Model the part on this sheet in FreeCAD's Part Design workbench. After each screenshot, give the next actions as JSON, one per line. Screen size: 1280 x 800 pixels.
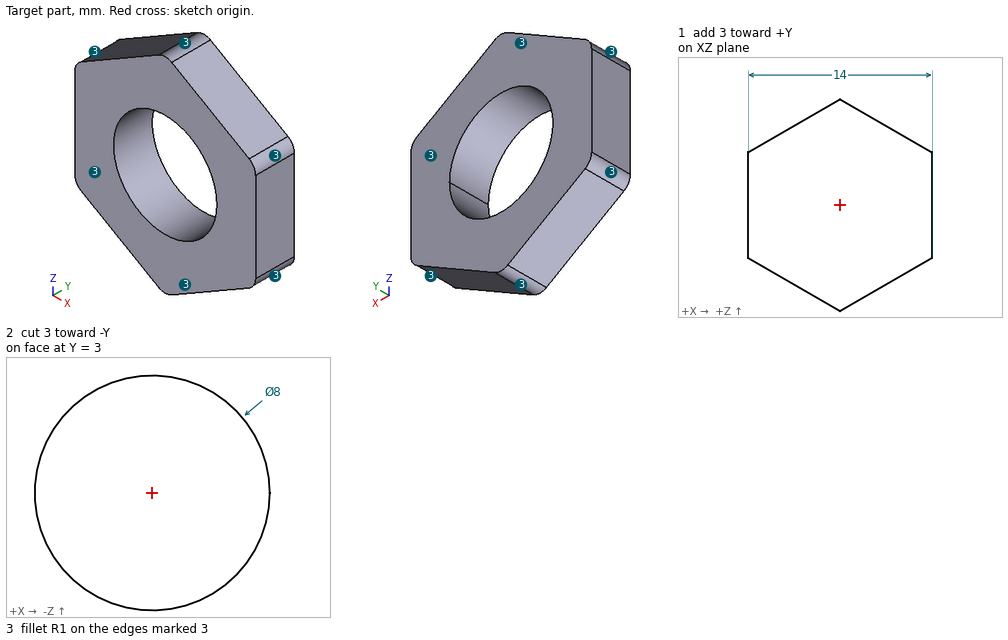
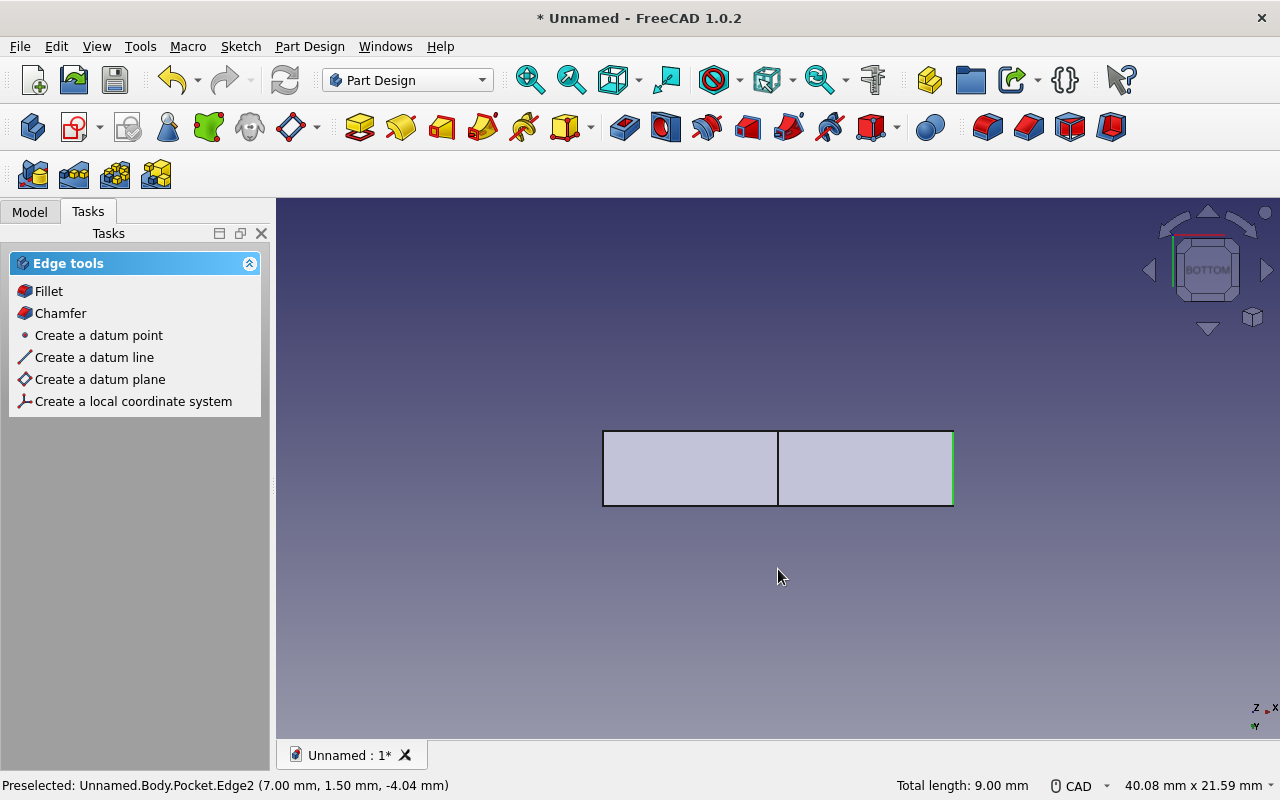
{"action": "key", "text": "v f"}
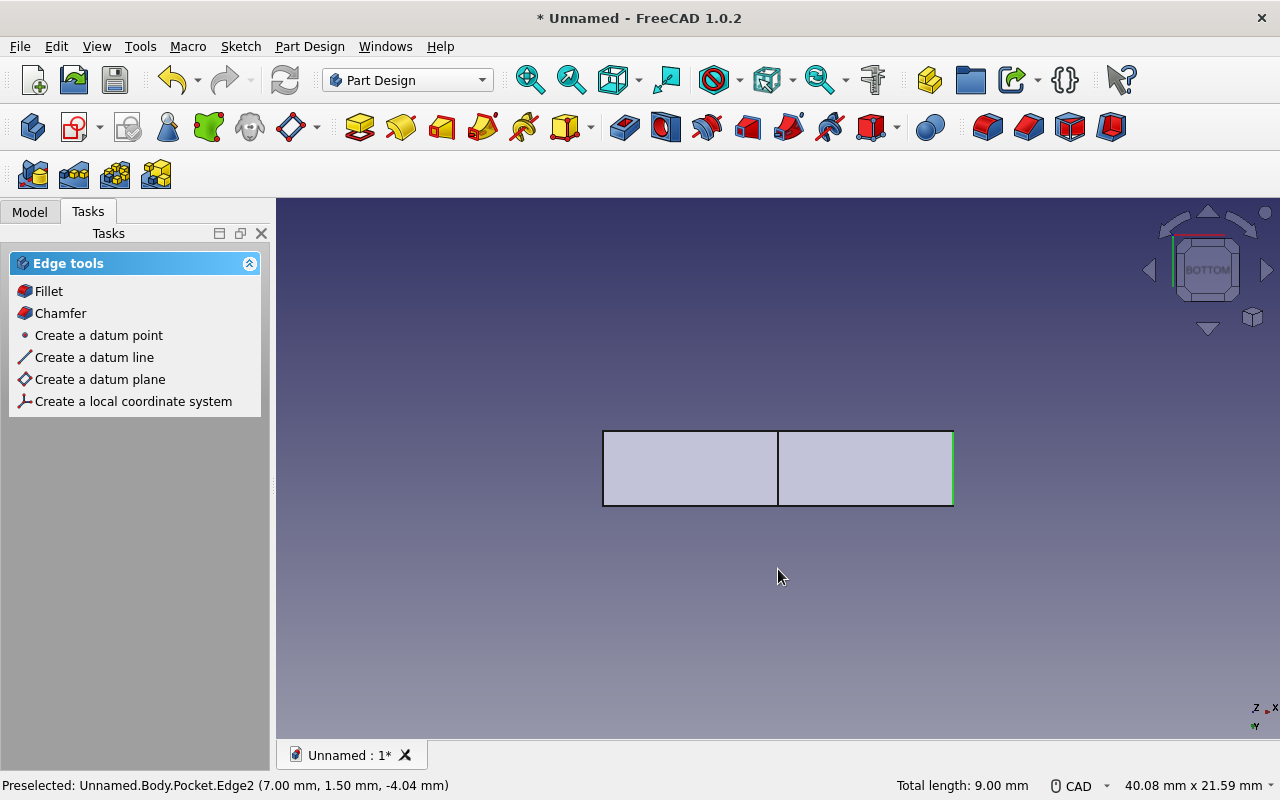
{"action": "left_click", "coordinate": [778, 467], "text": "ctrl"}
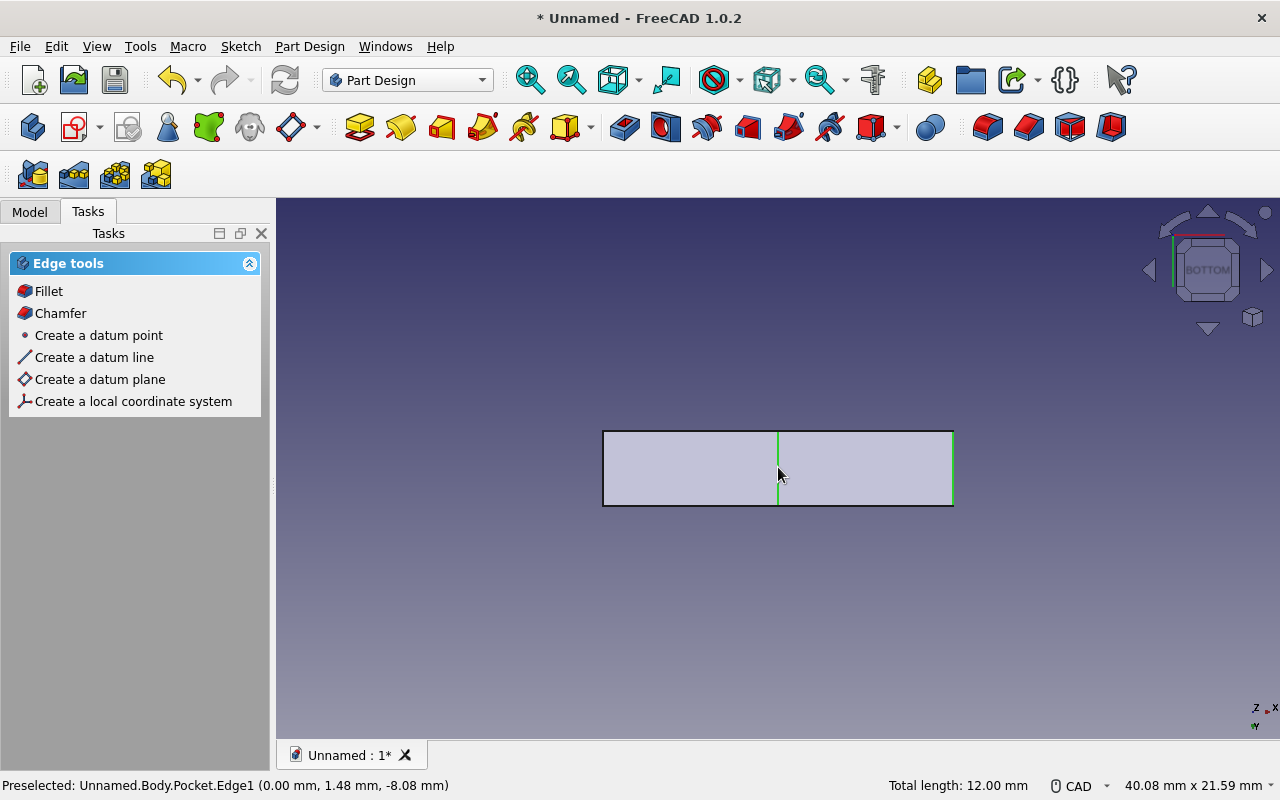
{"action": "key", "text": "4"}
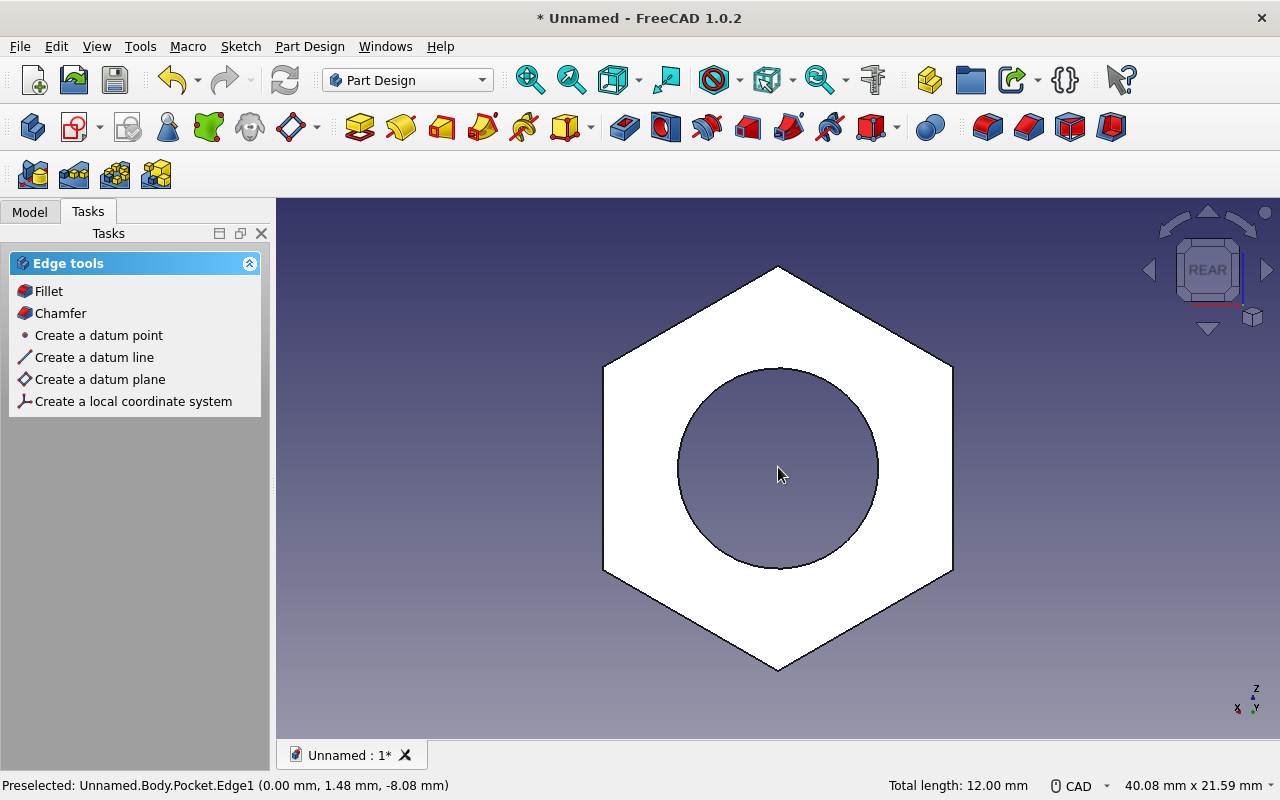
{"action": "key", "text": "6"}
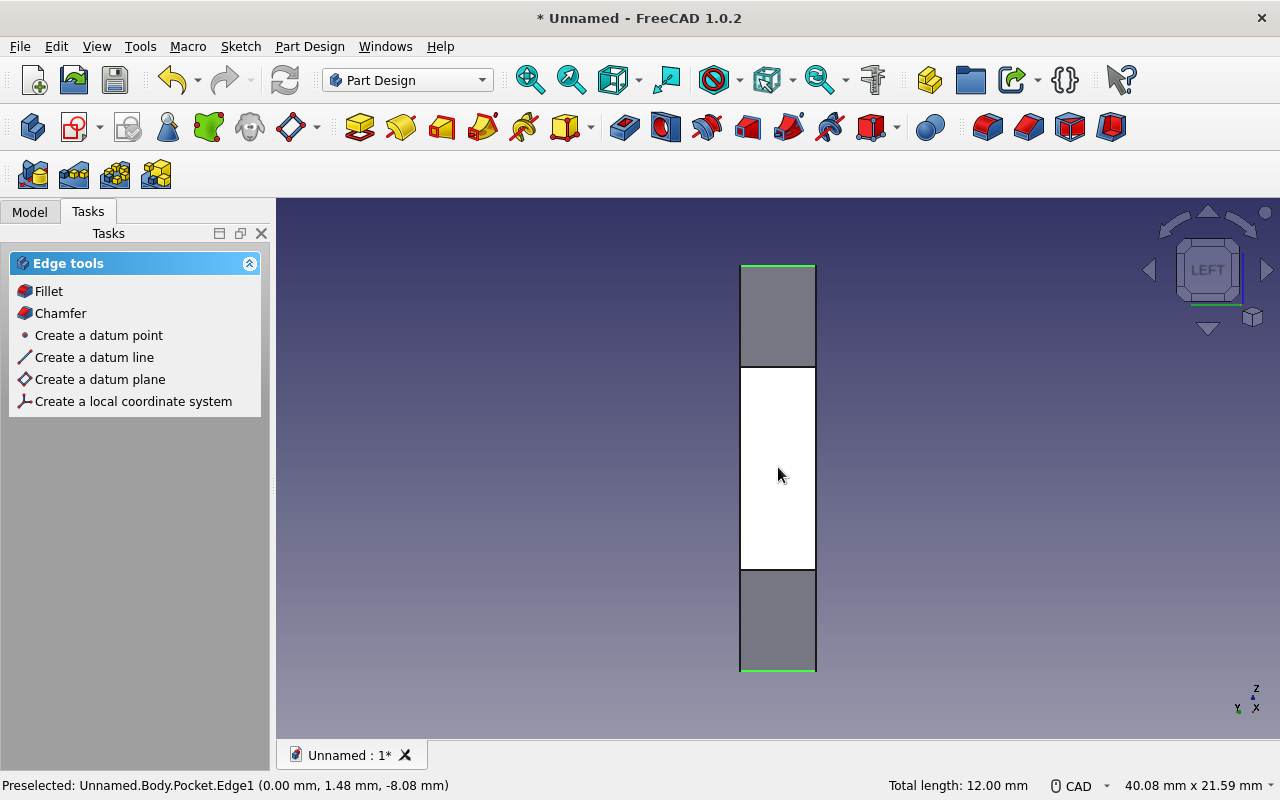
{"action": "left_click", "coordinate": [778, 366], "text": "ctrl"}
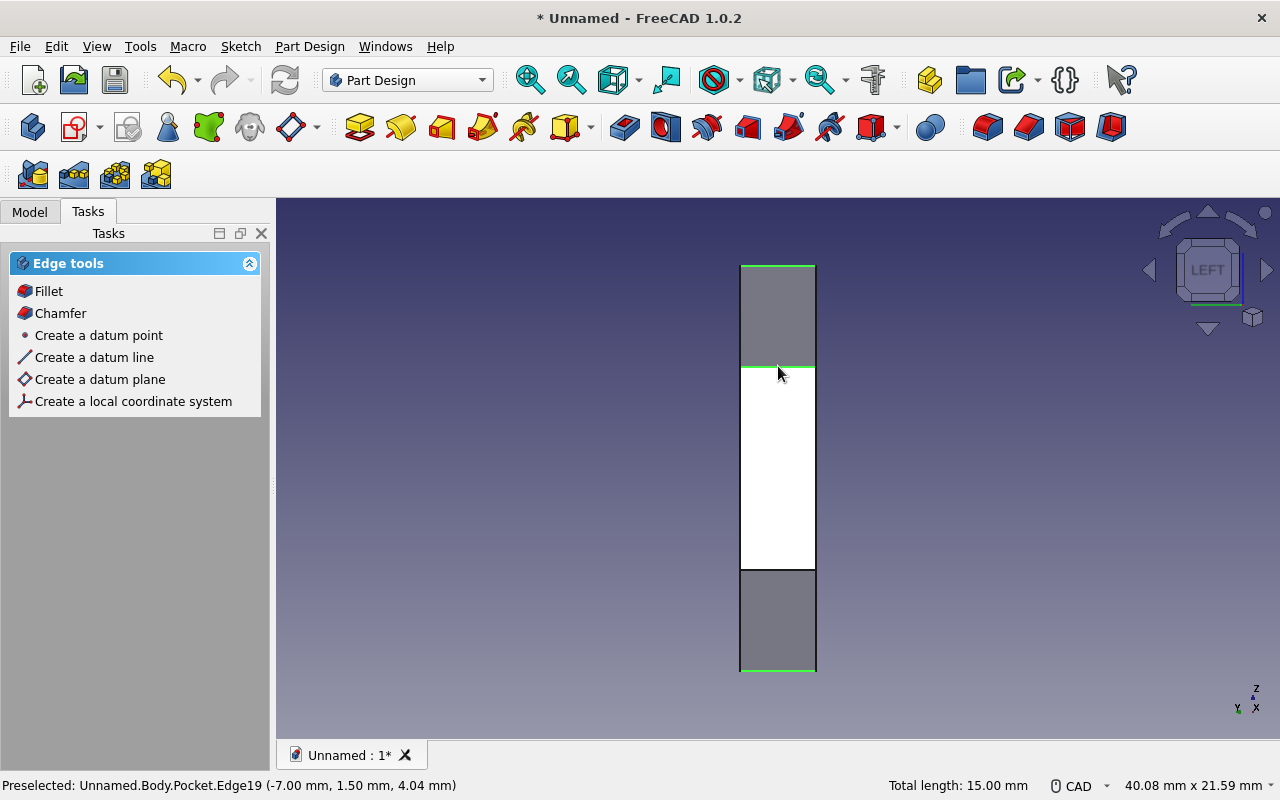
{"action": "left_click", "coordinate": [778, 569], "text": "ctrl"}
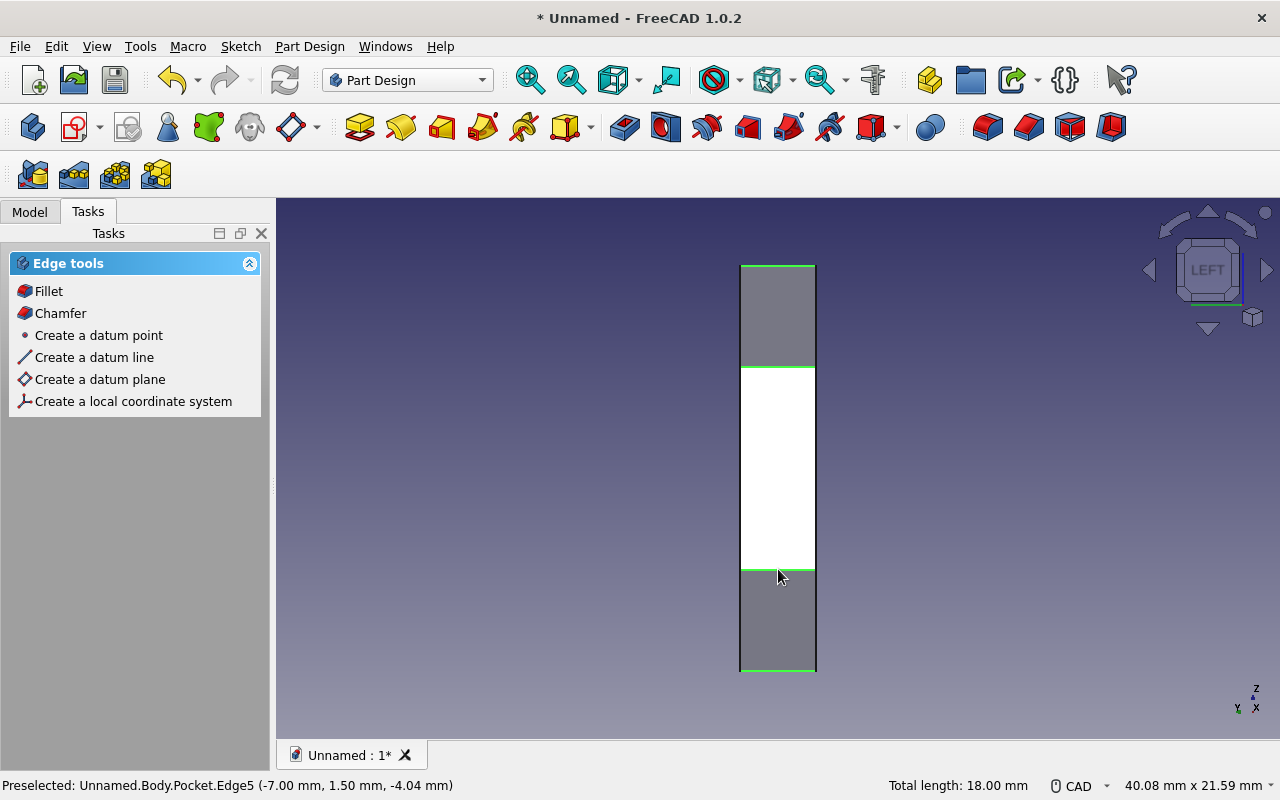
{"action": "left_click", "coordinate": [988, 128]}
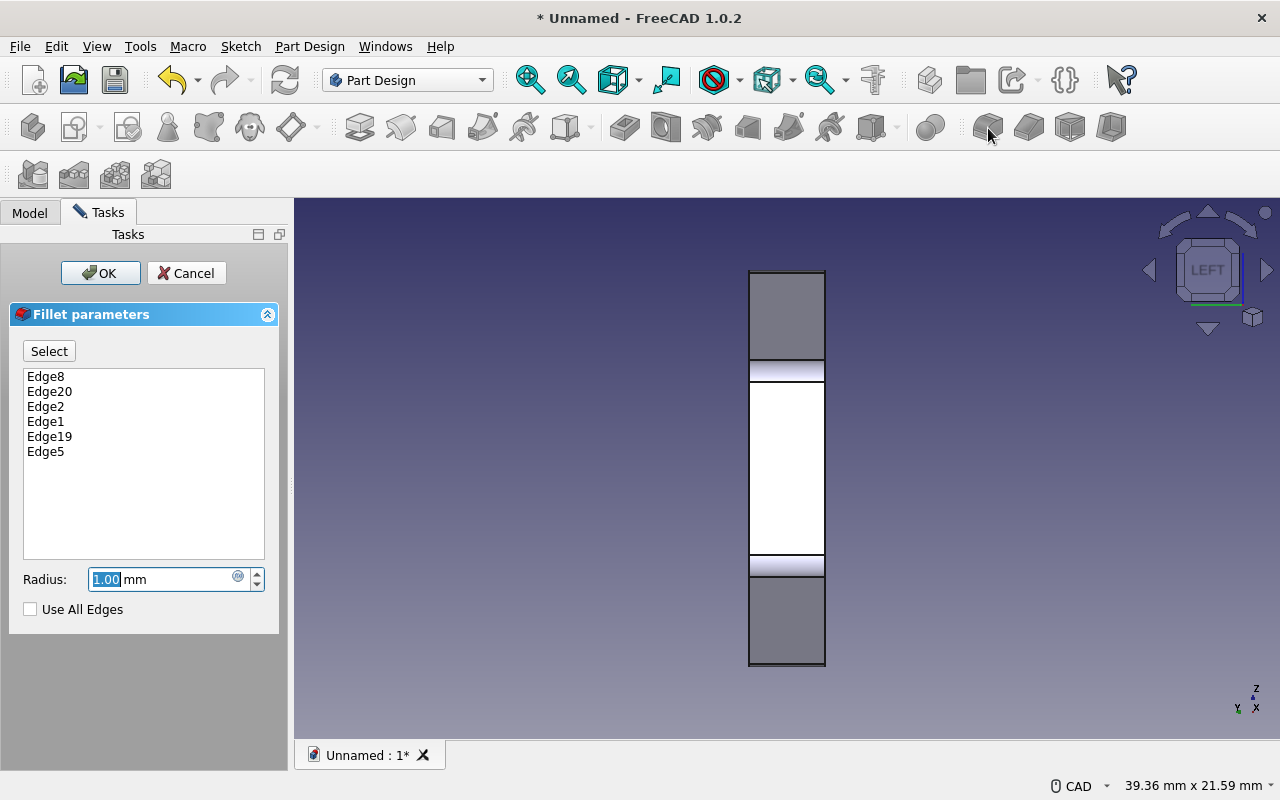
{"action": "type", "text": "1"}
{"action": "key", "text": "Tab"}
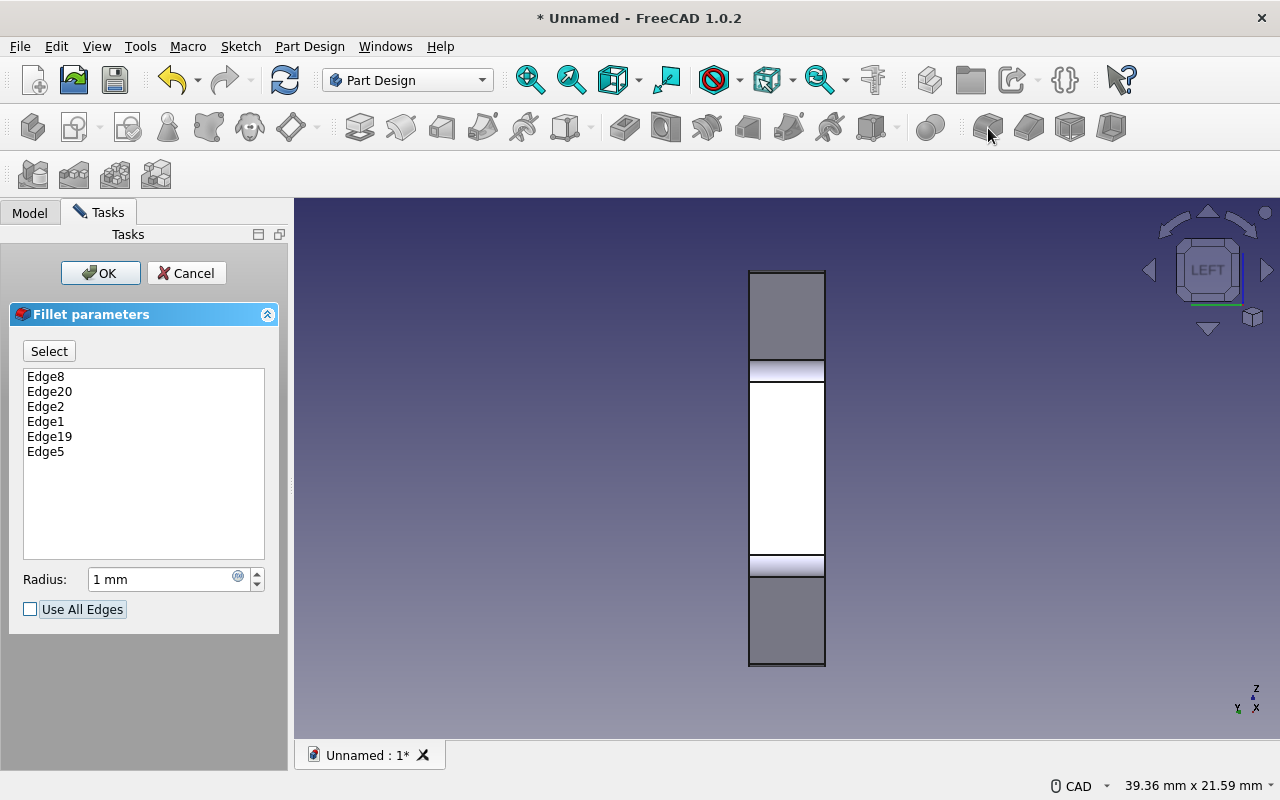
{"action": "left_click", "coordinate": [101, 273]}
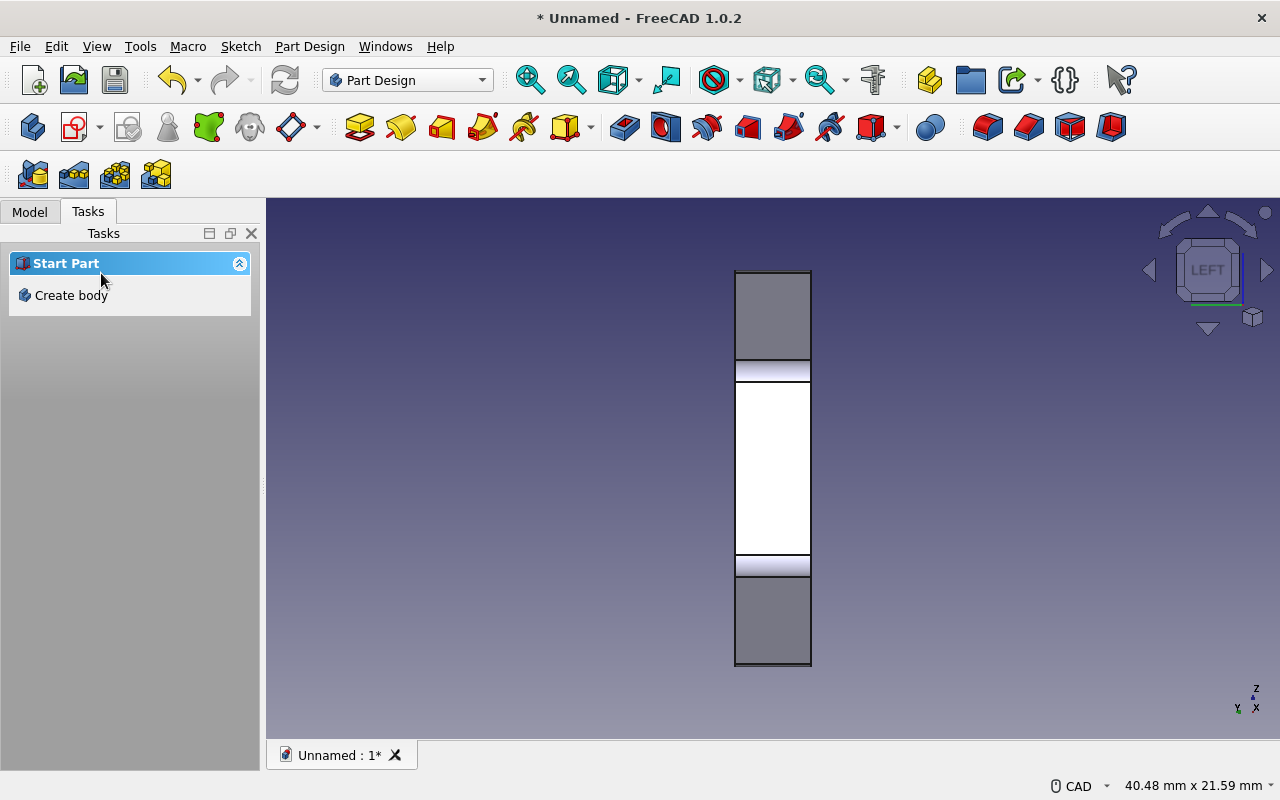
{"action": "key", "text": "0"}